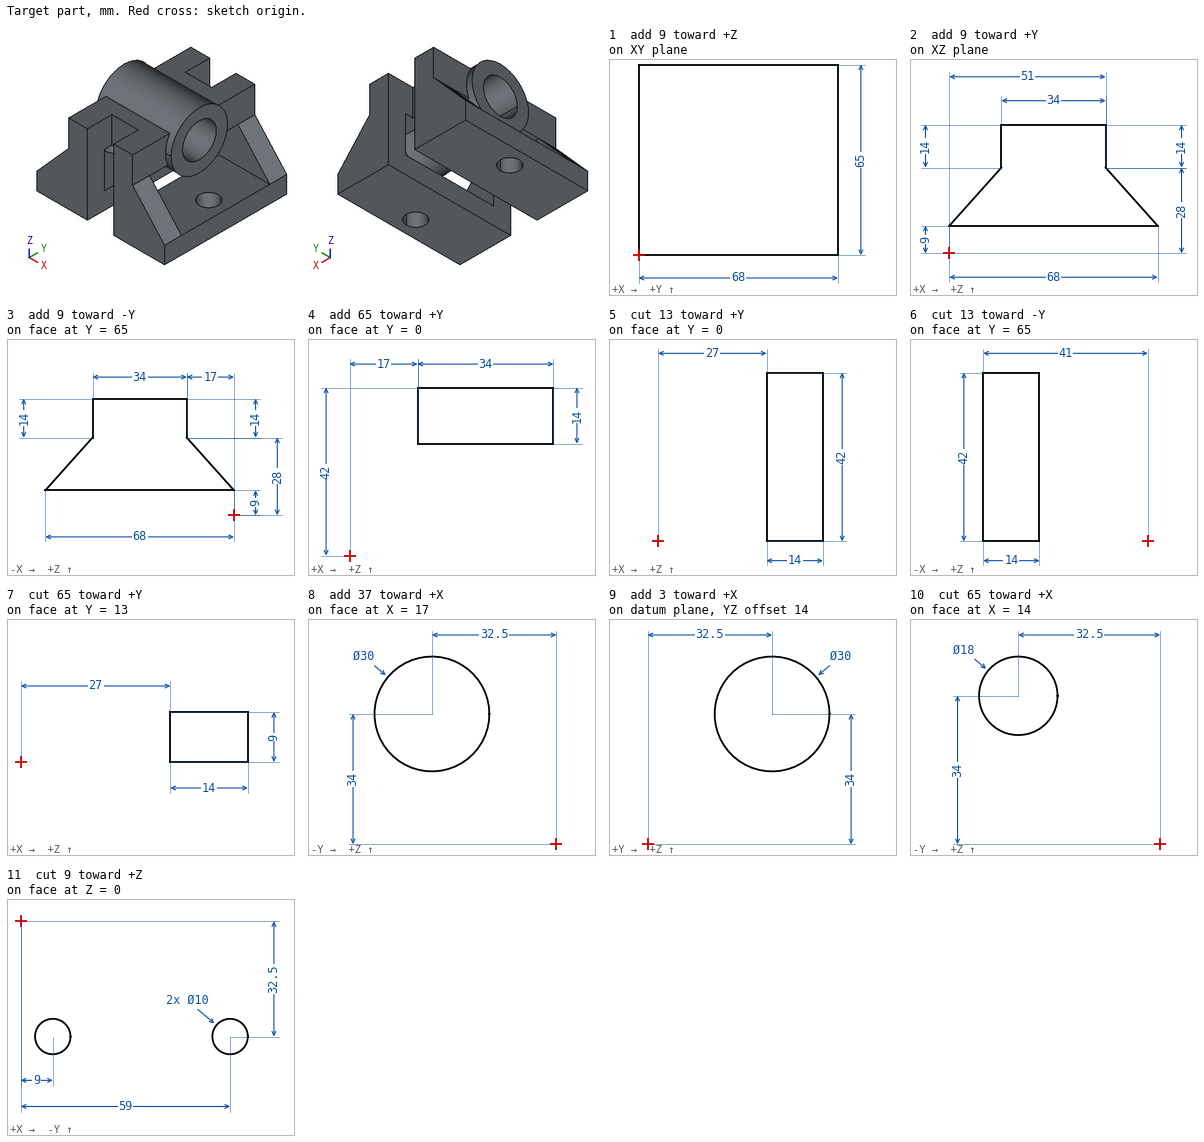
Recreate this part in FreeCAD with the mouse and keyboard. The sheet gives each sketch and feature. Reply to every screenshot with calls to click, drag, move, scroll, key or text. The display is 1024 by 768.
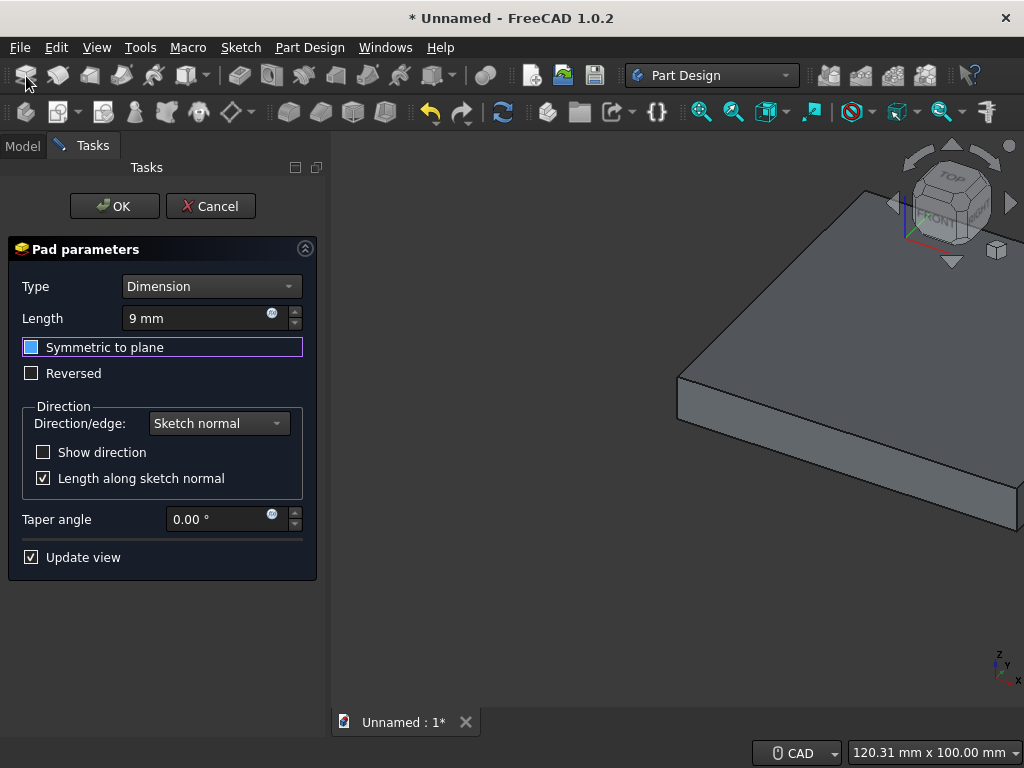
click(115, 206)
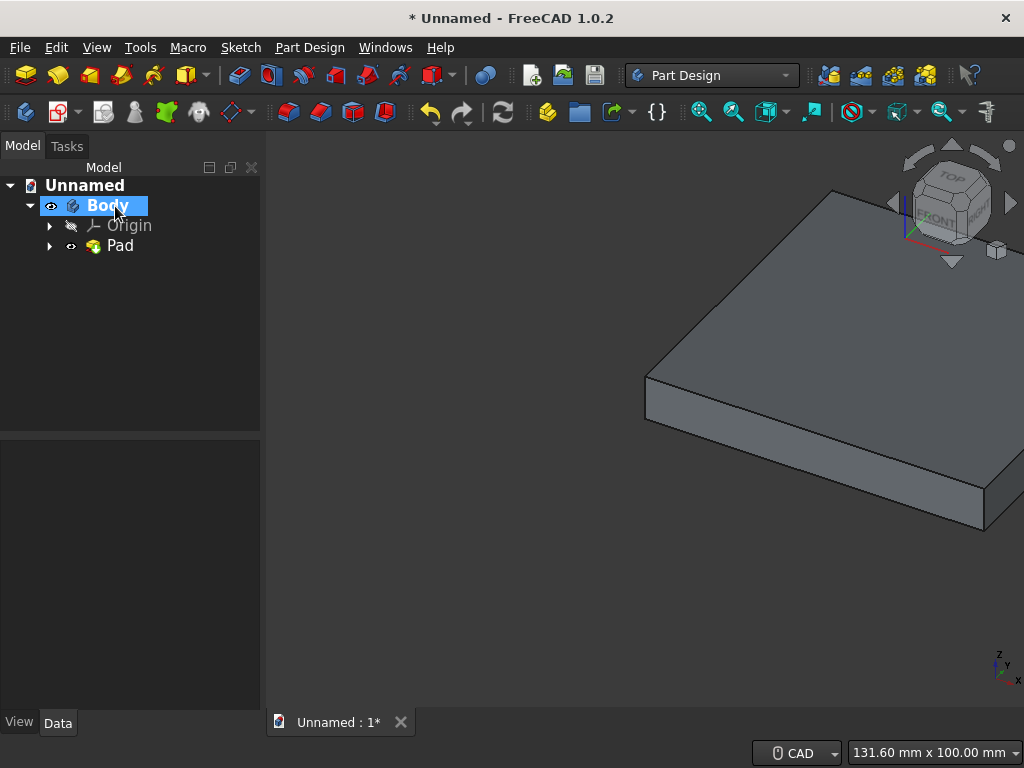
key(v)
key(f)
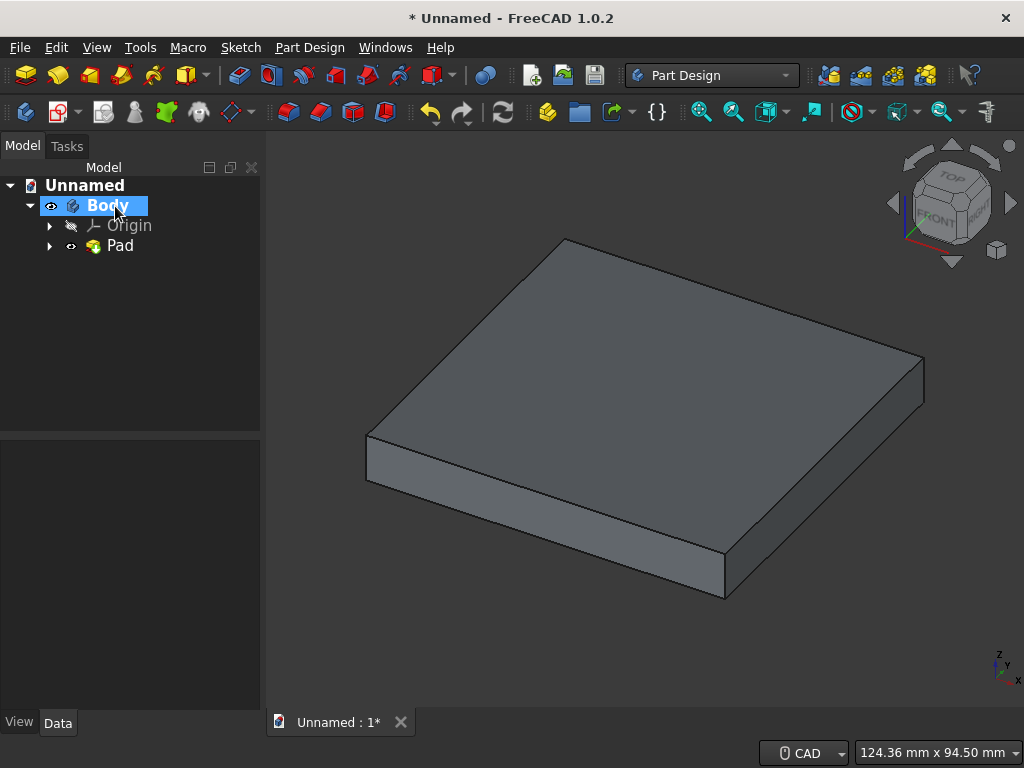
click(58, 112)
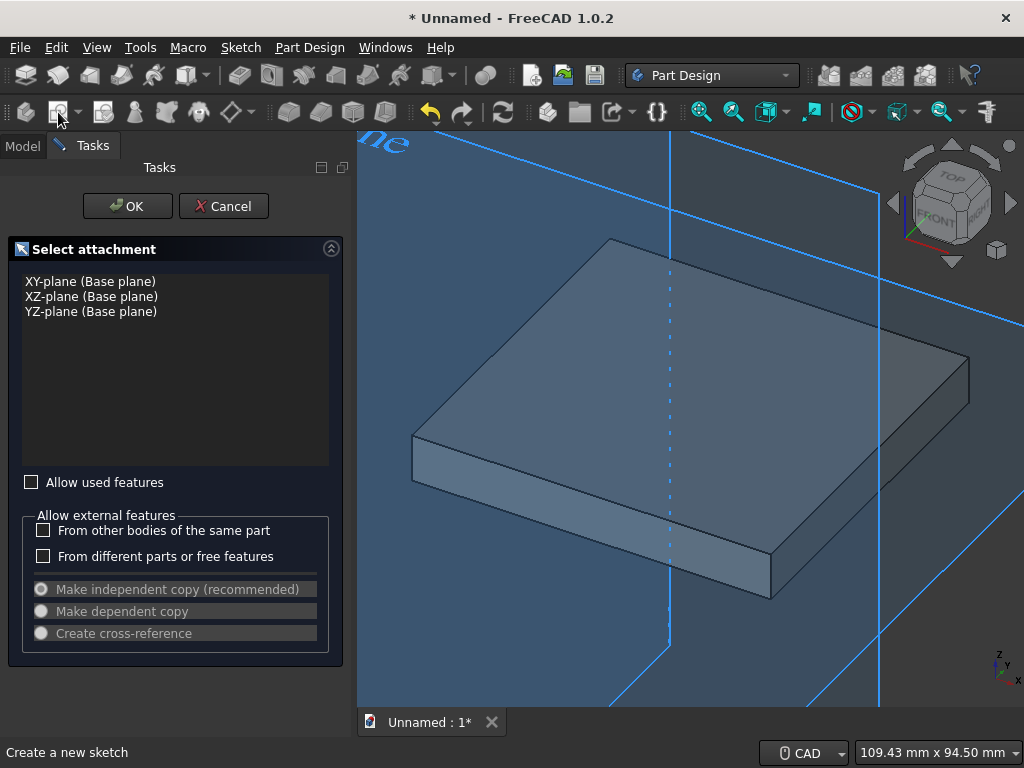
click(82, 296)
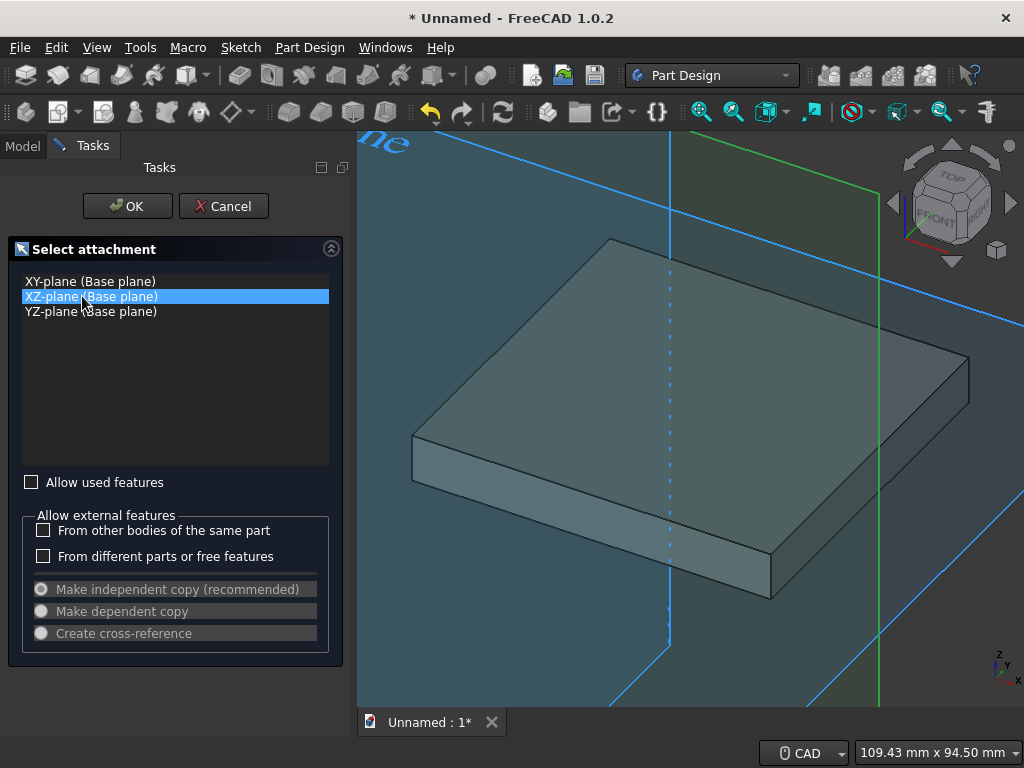
click(128, 206)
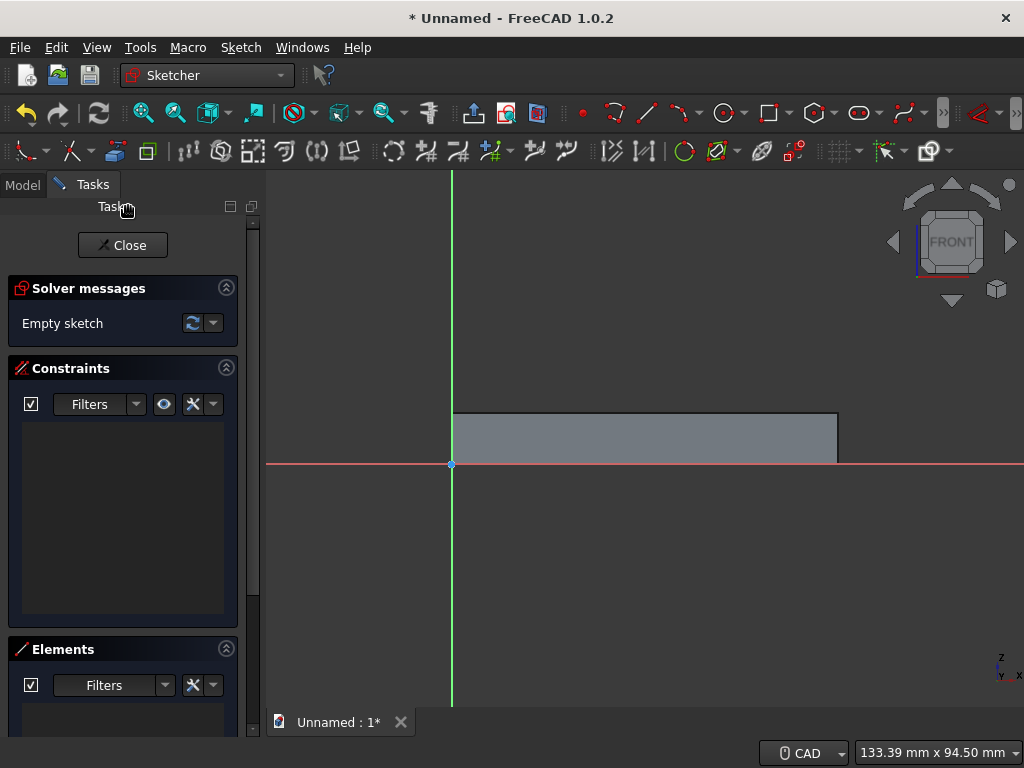
scroll(294, 679, down, 1)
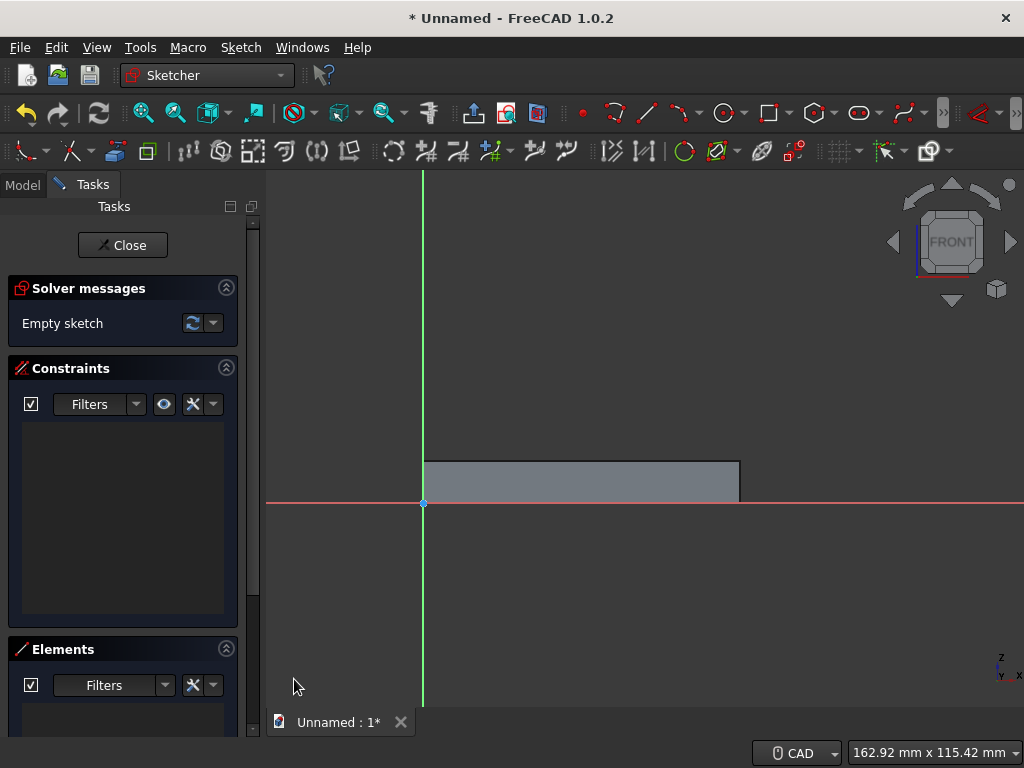
click(616, 114)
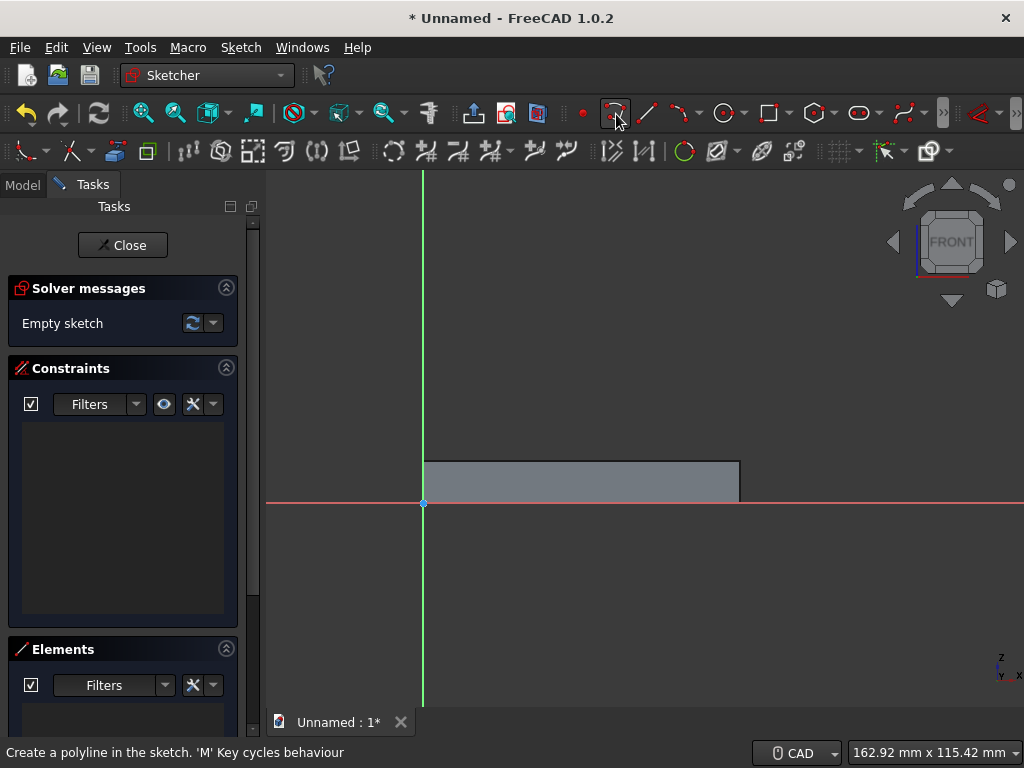
click(423, 461)
click(740, 461)
click(660, 373)
click(660, 308)
click(502, 308)
click(502, 373)
click(423, 462)
key(Escape)
key(Escape)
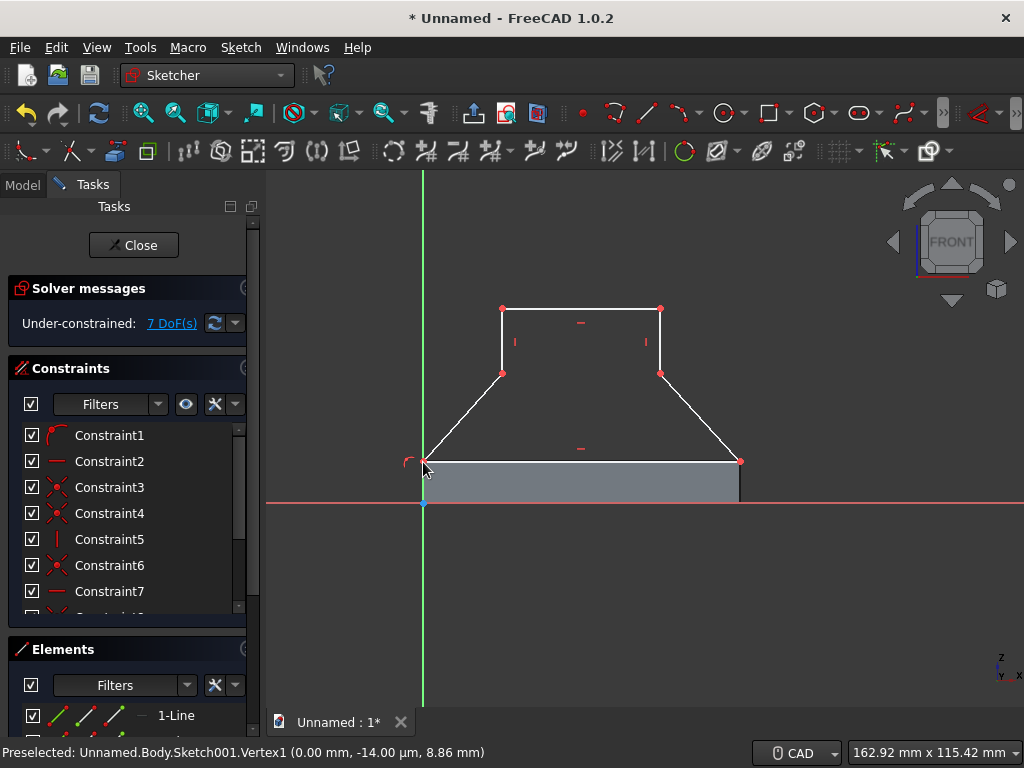
click(978, 114)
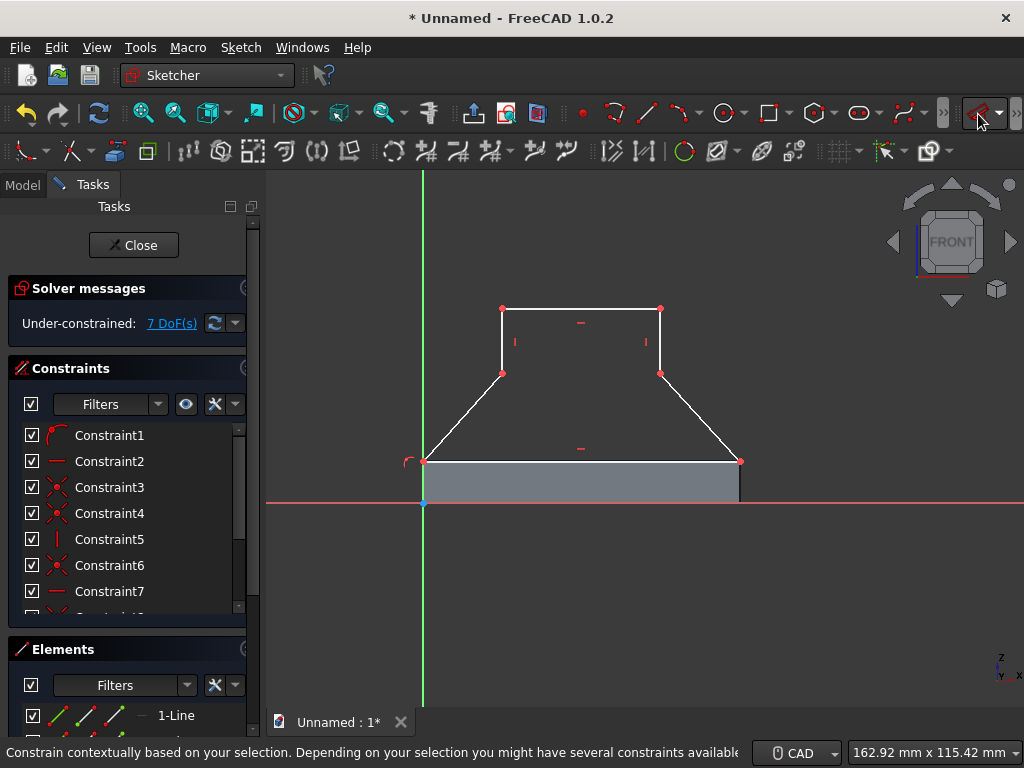
click(518, 462)
click(582, 428)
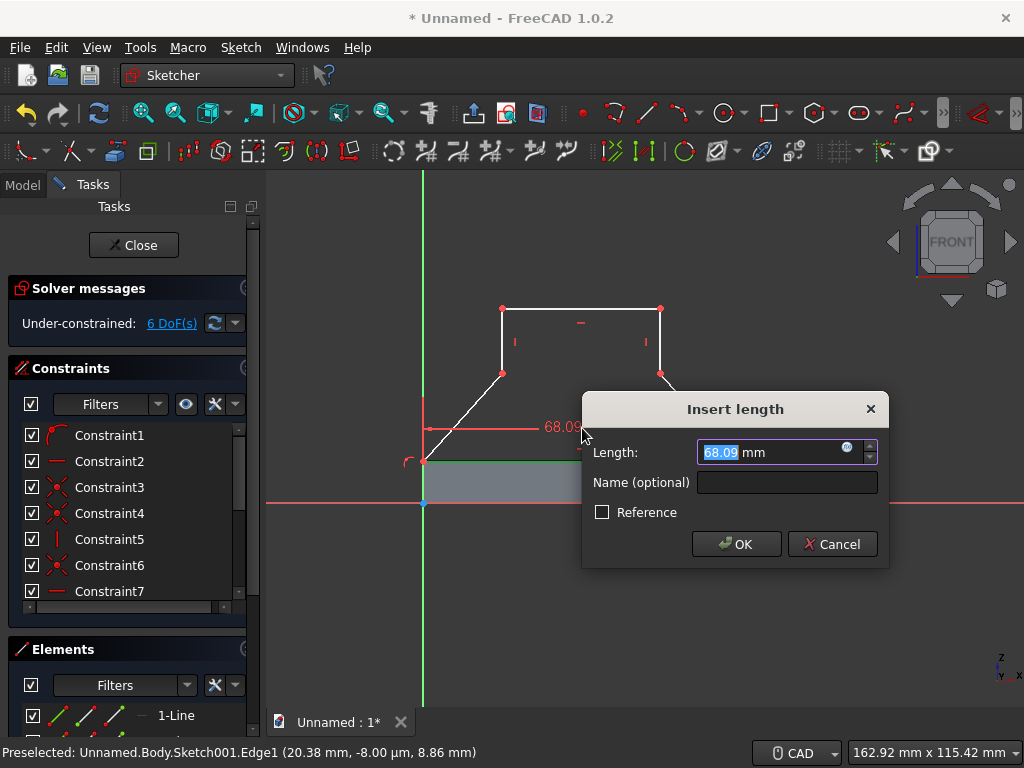
text(68)
key(Return)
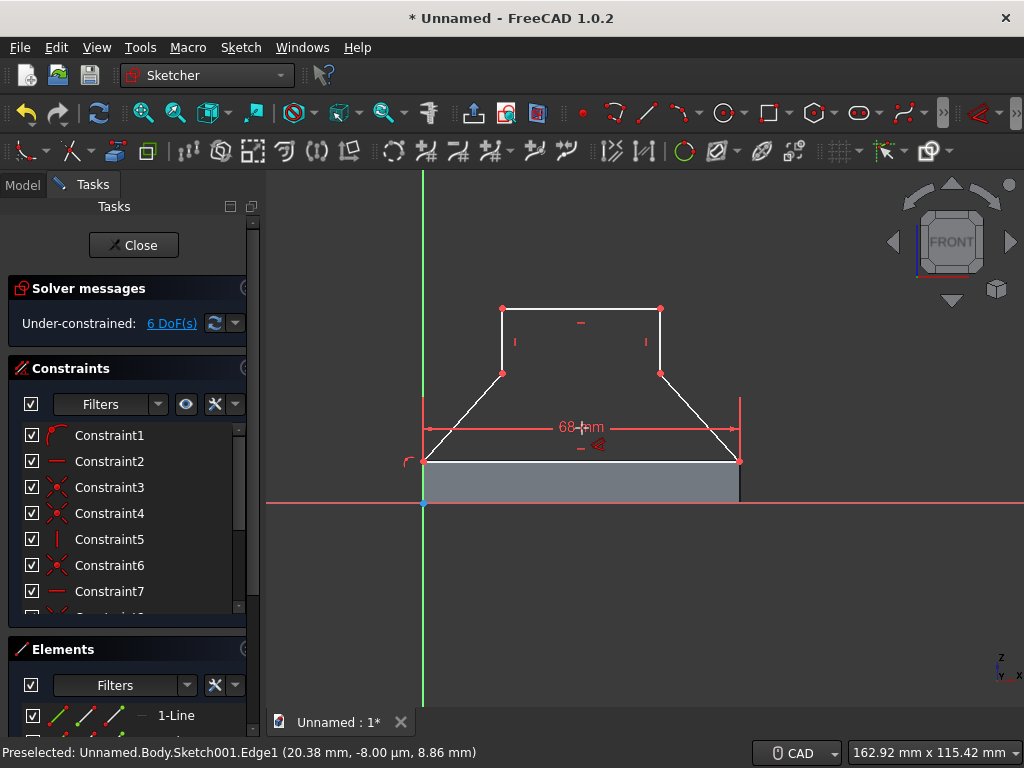
click(660, 355)
click(694, 342)